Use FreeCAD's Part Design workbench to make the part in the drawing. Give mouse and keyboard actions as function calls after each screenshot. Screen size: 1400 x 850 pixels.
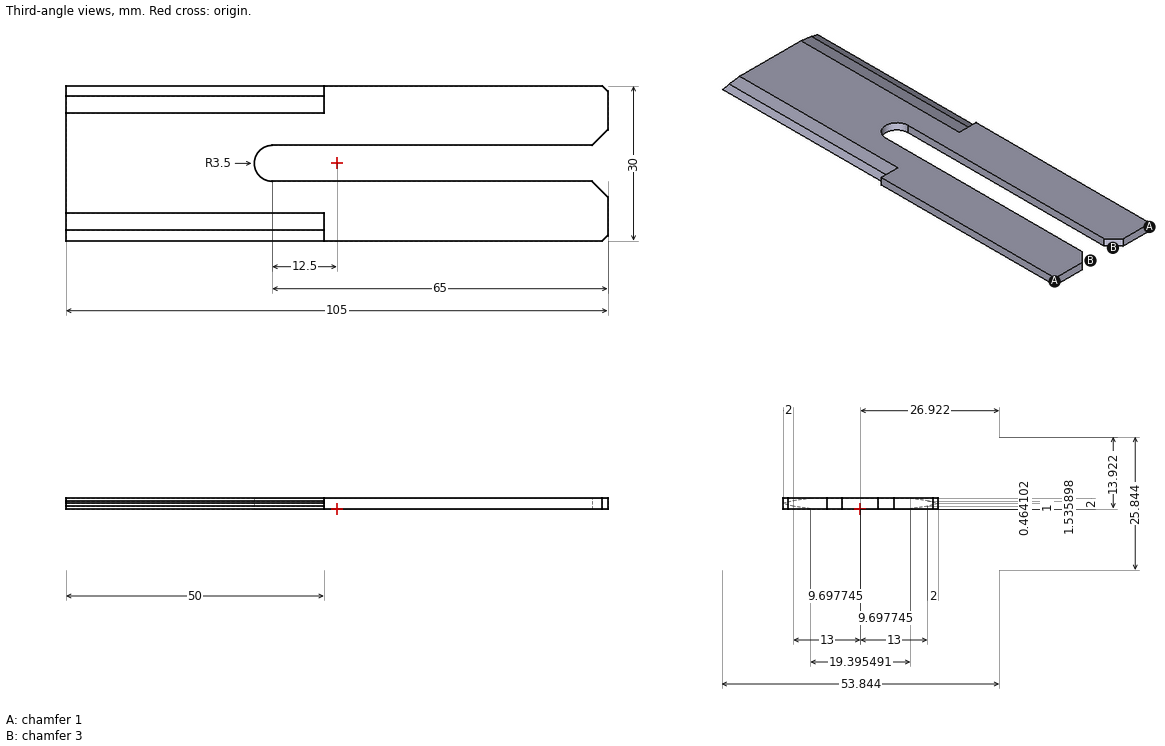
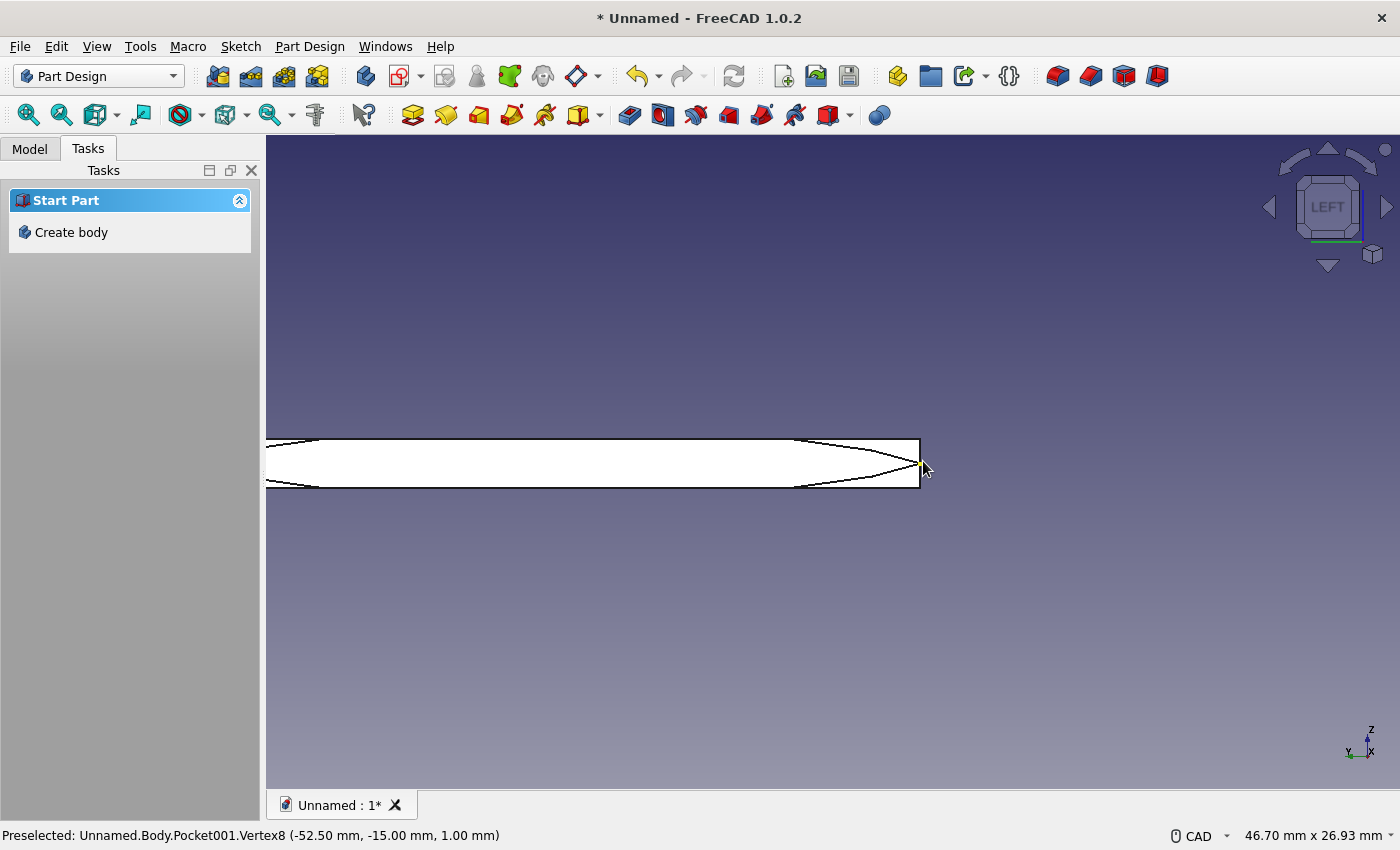
click(29, 116)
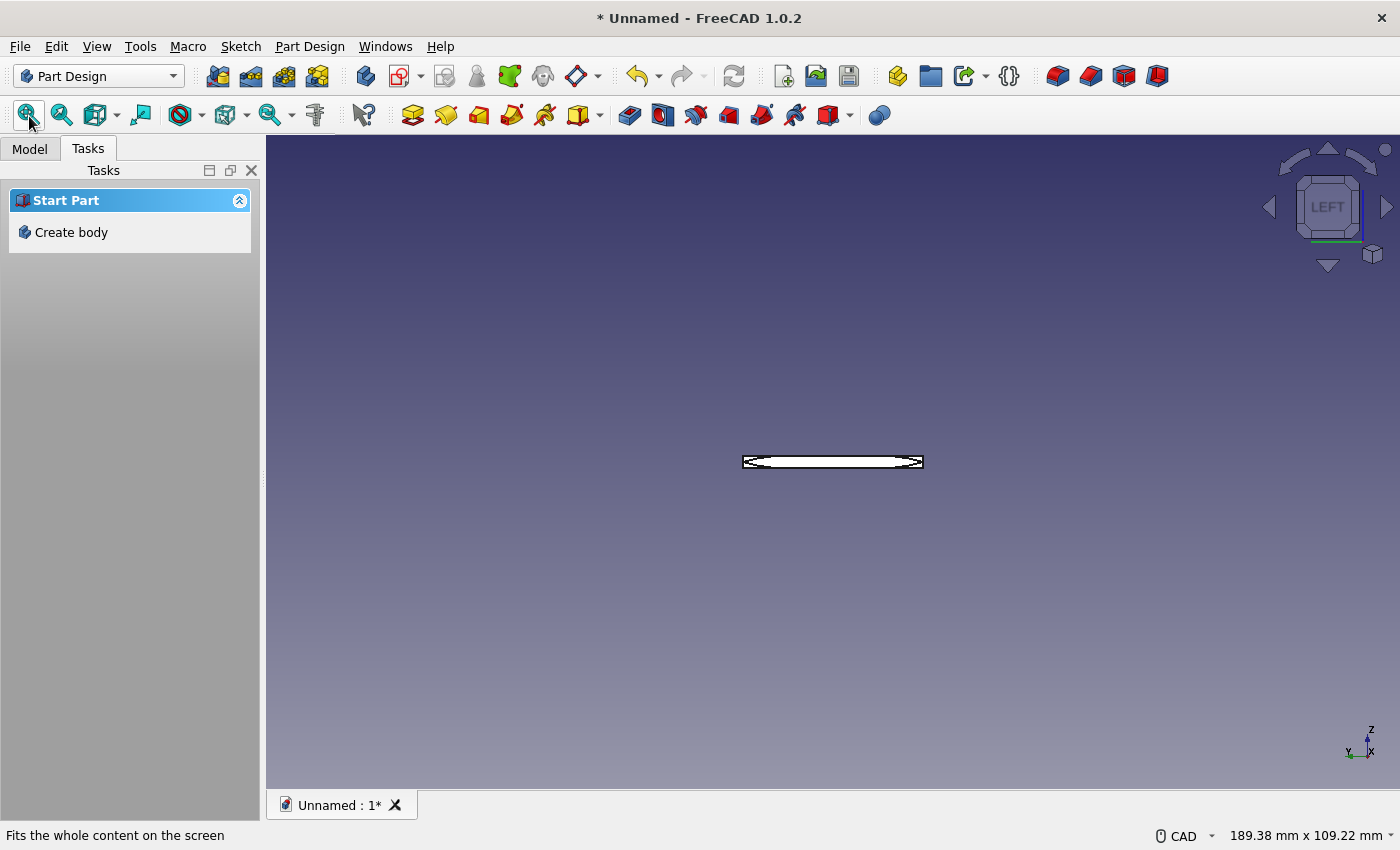
key(0)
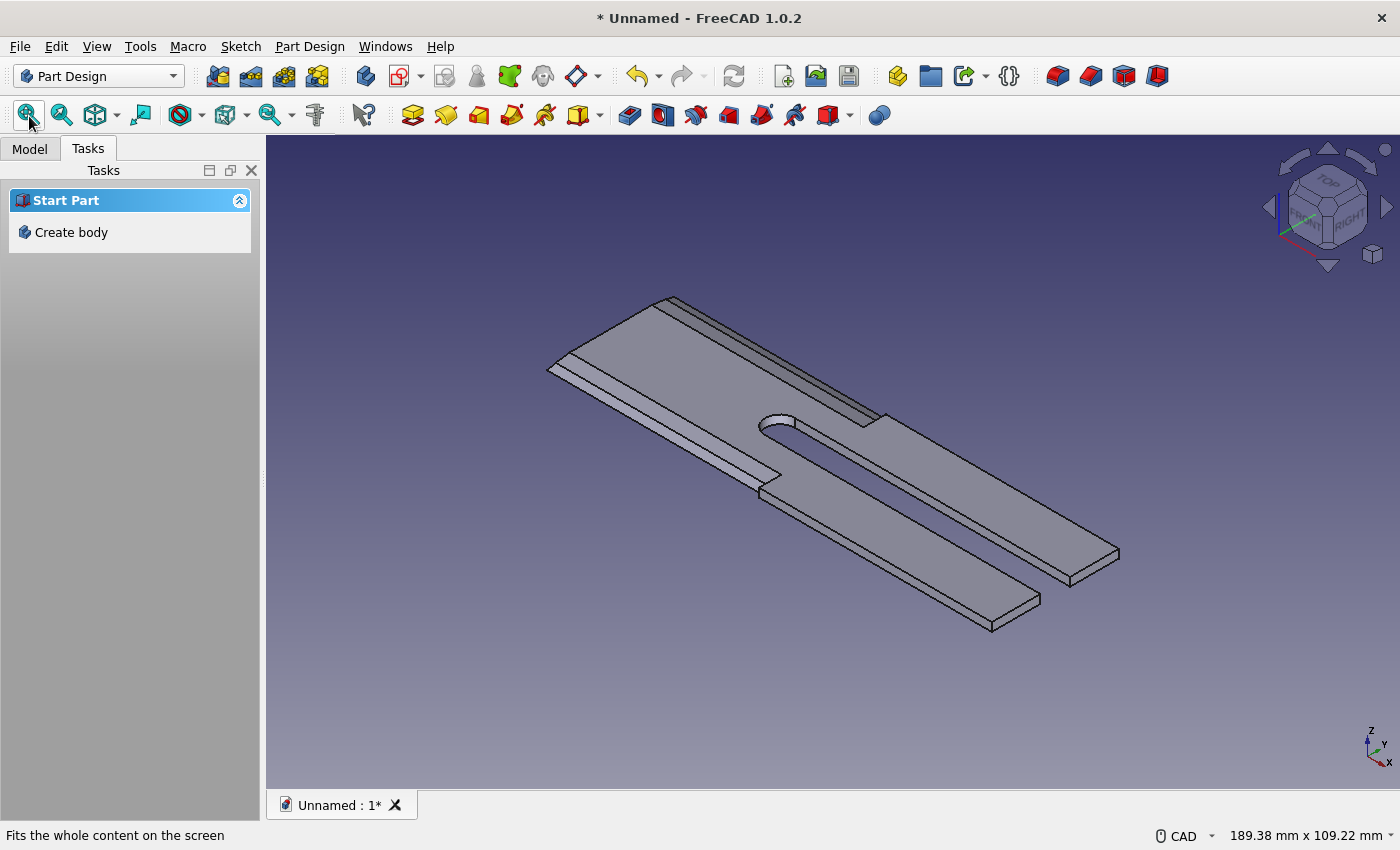
click(992, 628)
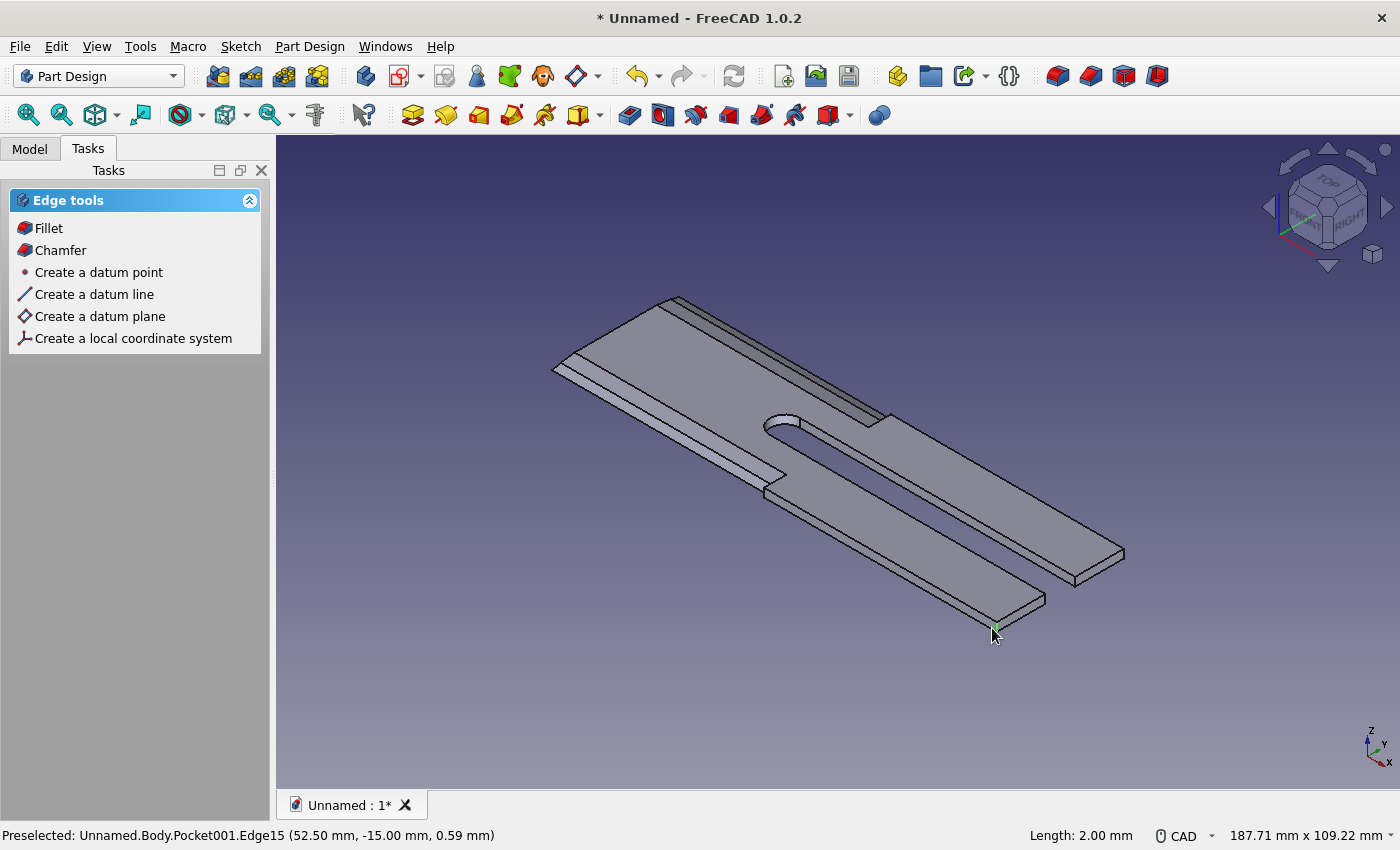
scroll(1124, 553, up, 7)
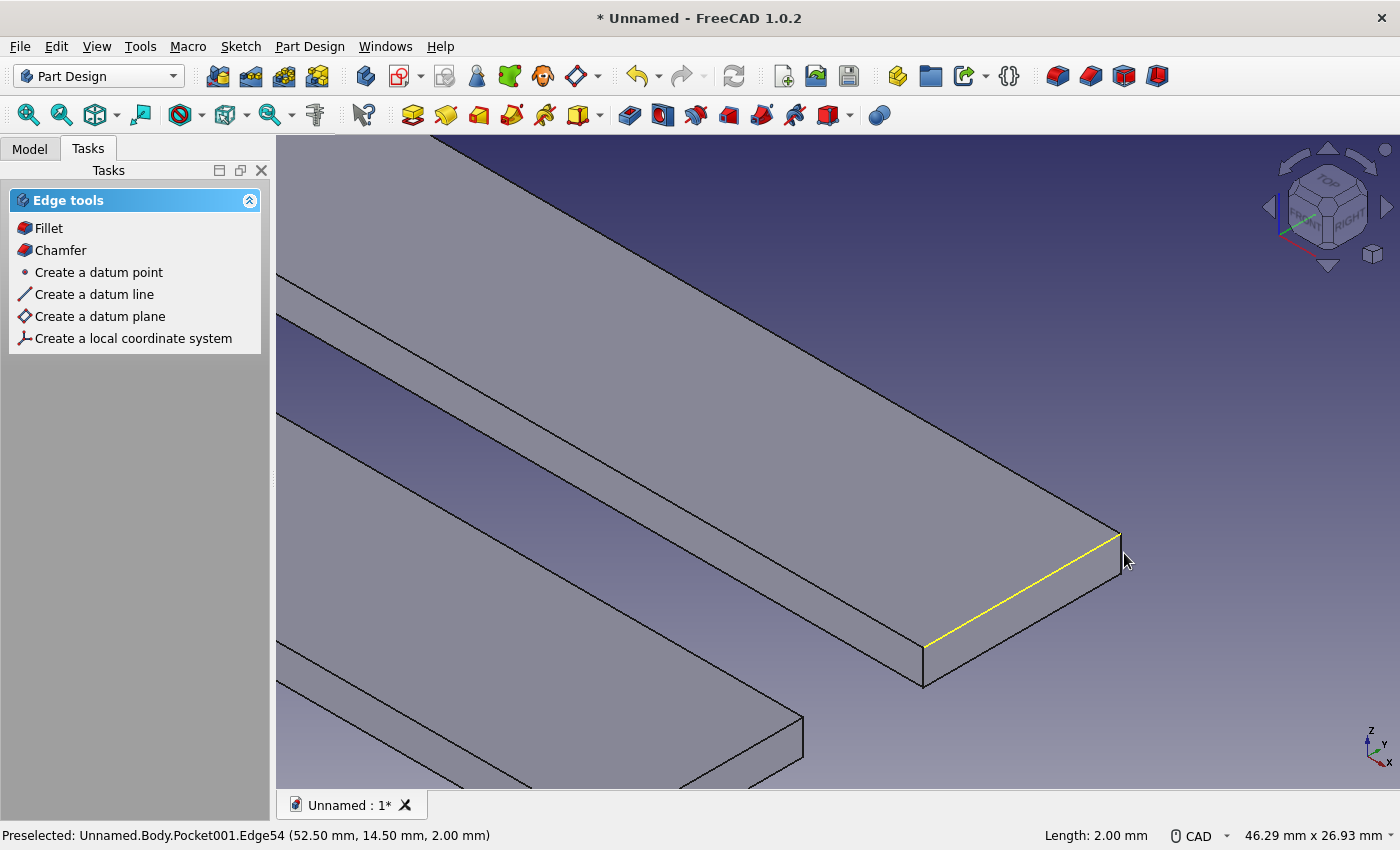
click(29, 116)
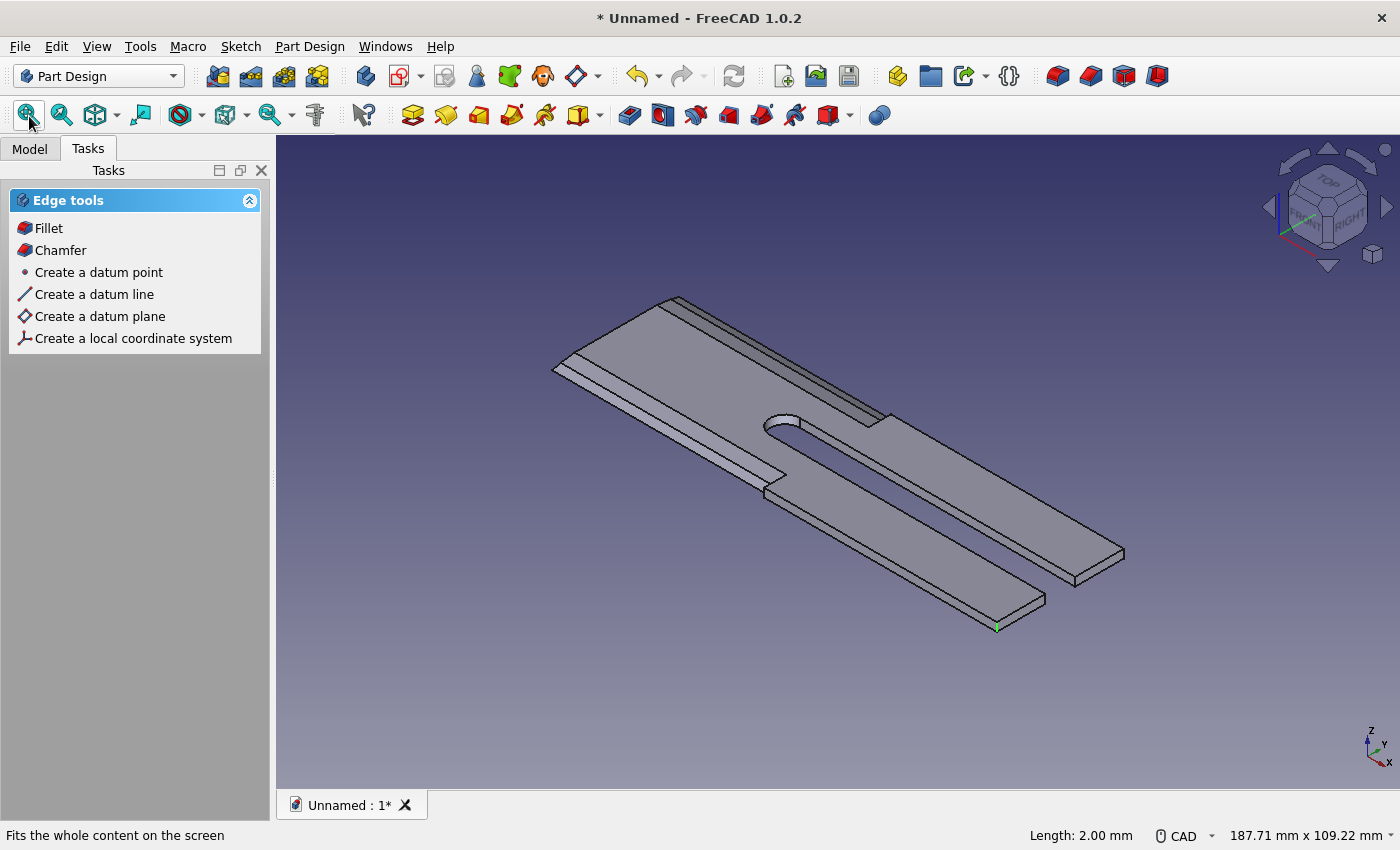
key(2)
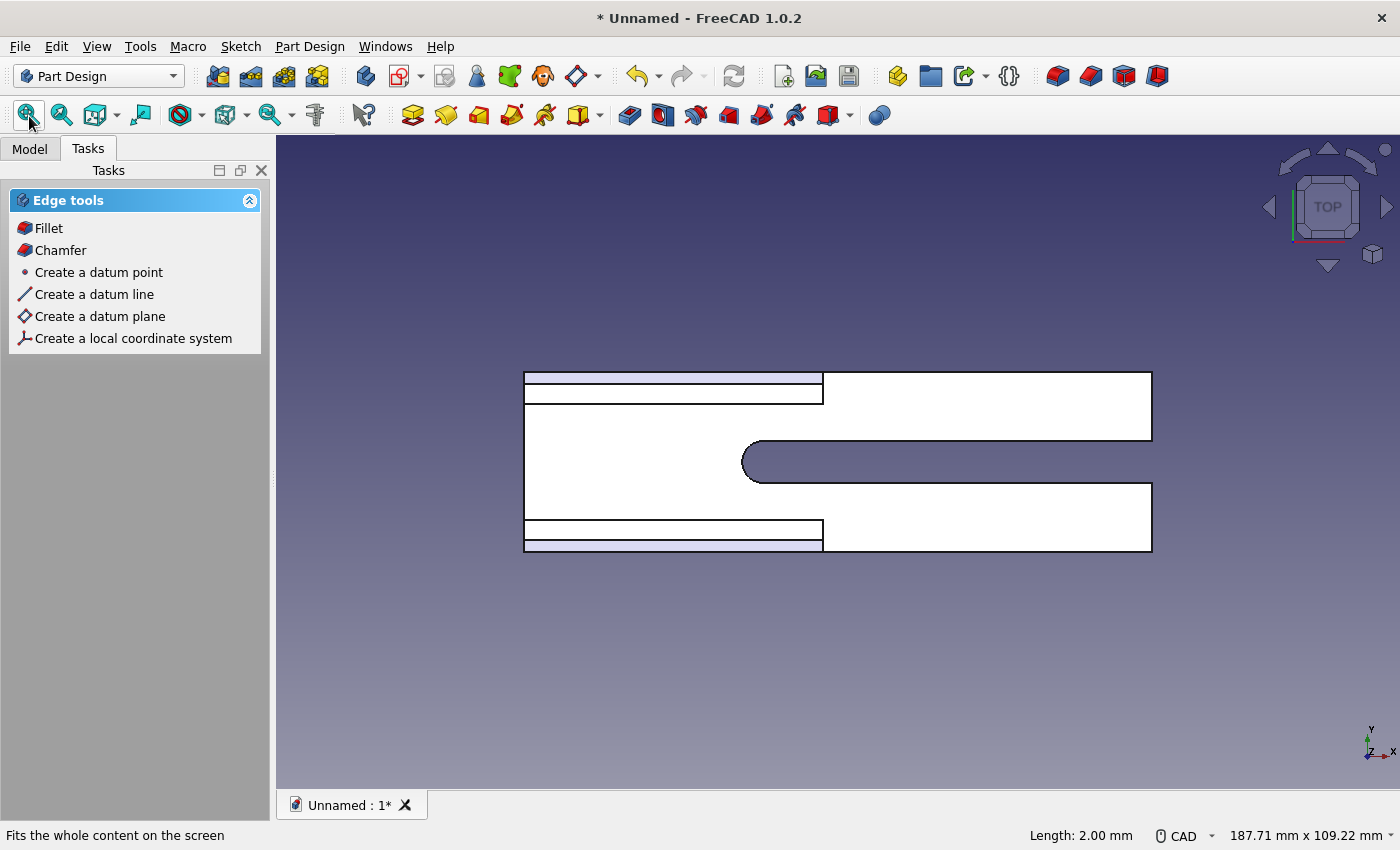
scroll(1152, 371, up, 7)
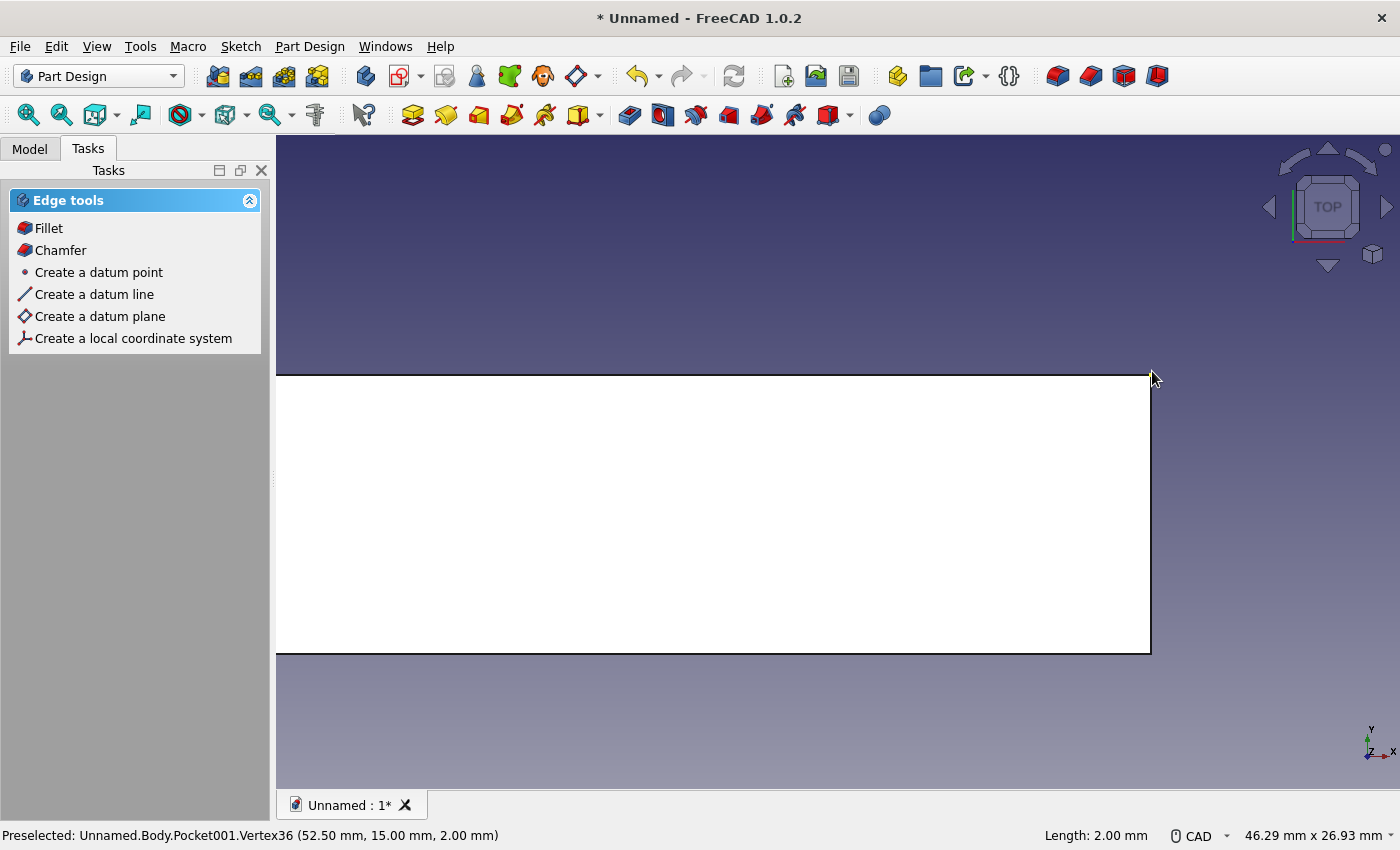
click(29, 116)